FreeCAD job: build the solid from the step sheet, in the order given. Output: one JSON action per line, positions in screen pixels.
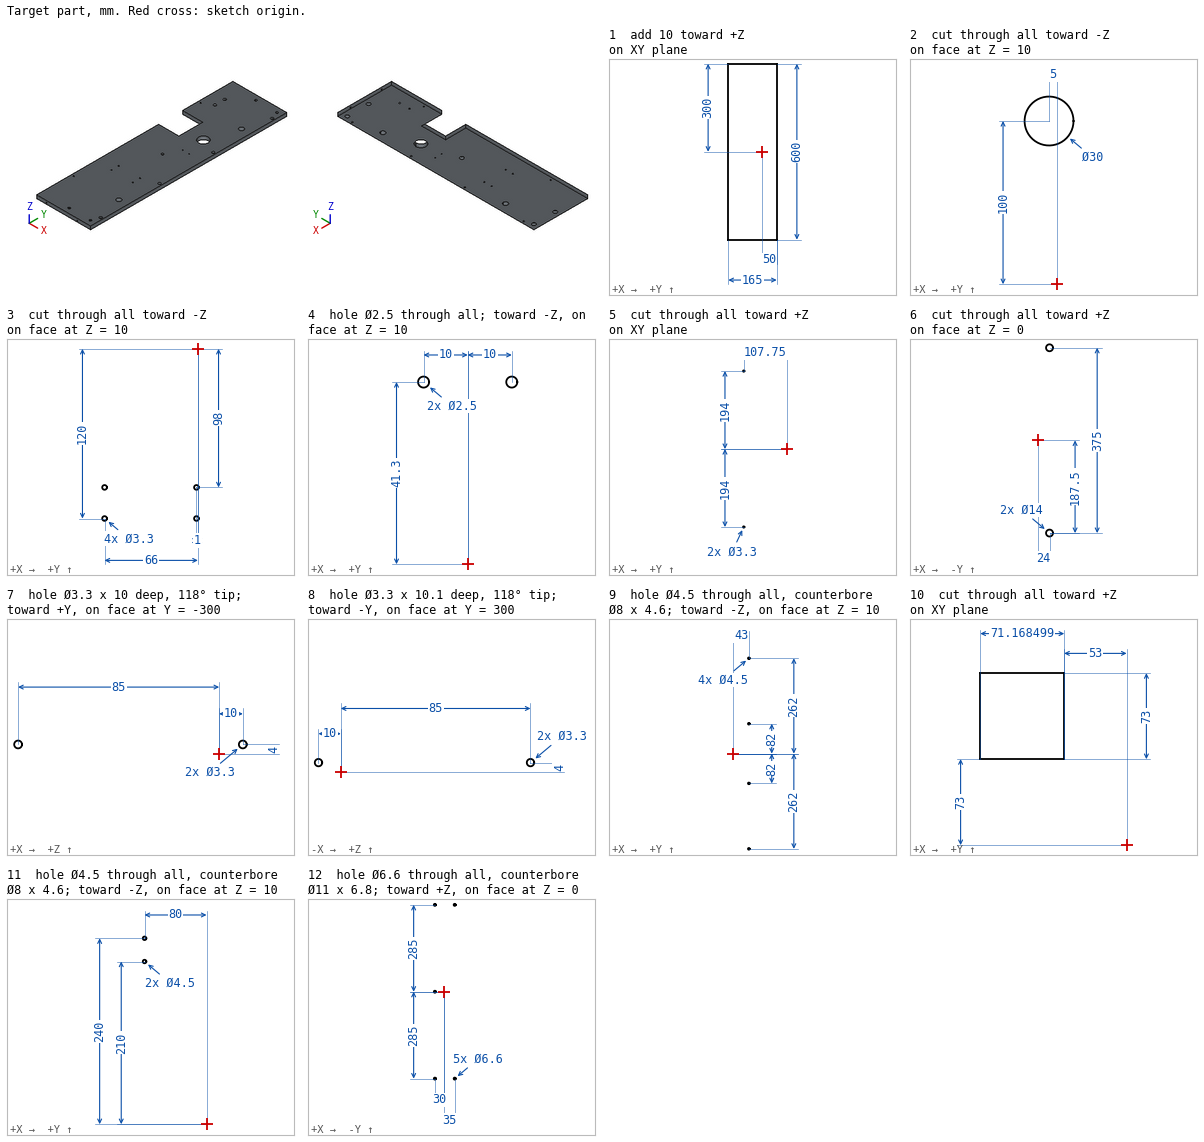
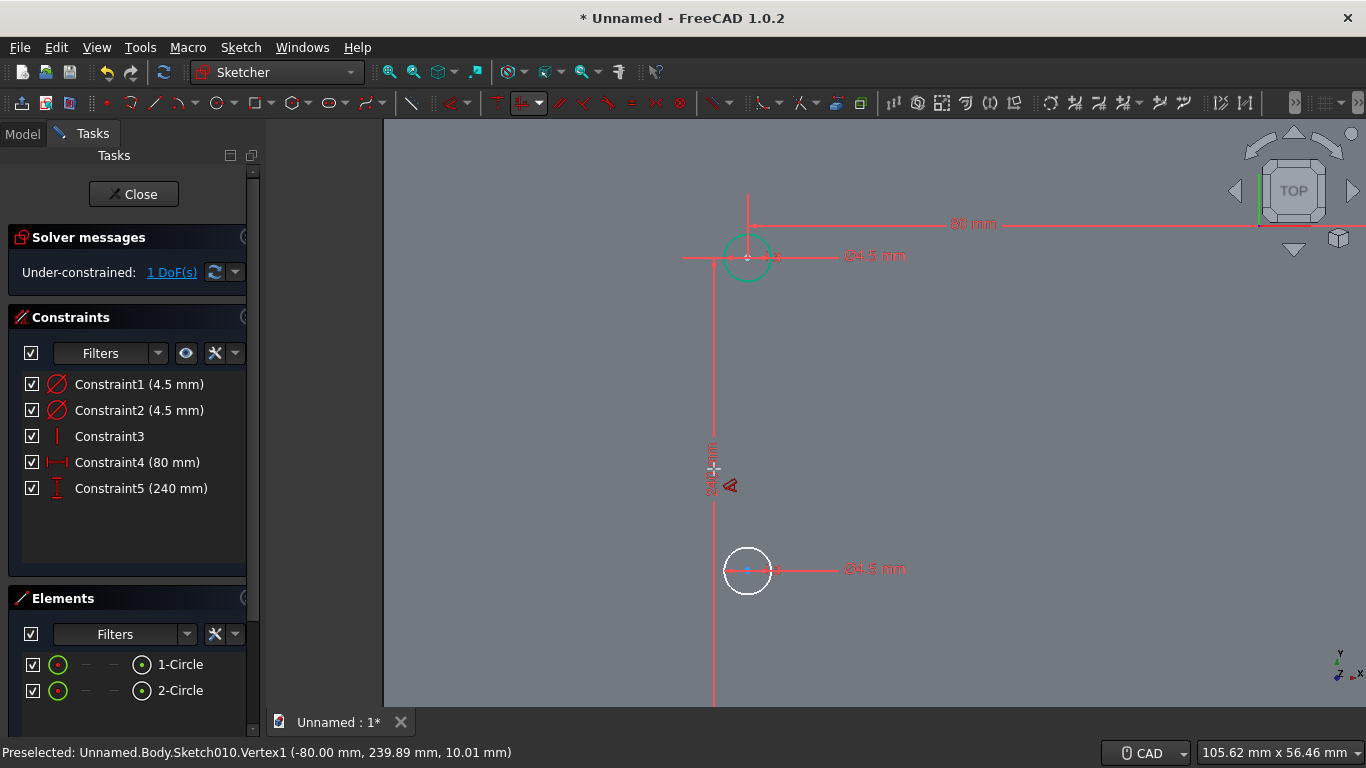
{"action": "left_click", "coordinate": [748, 571]}
{"action": "left_click", "coordinate": [714, 625]}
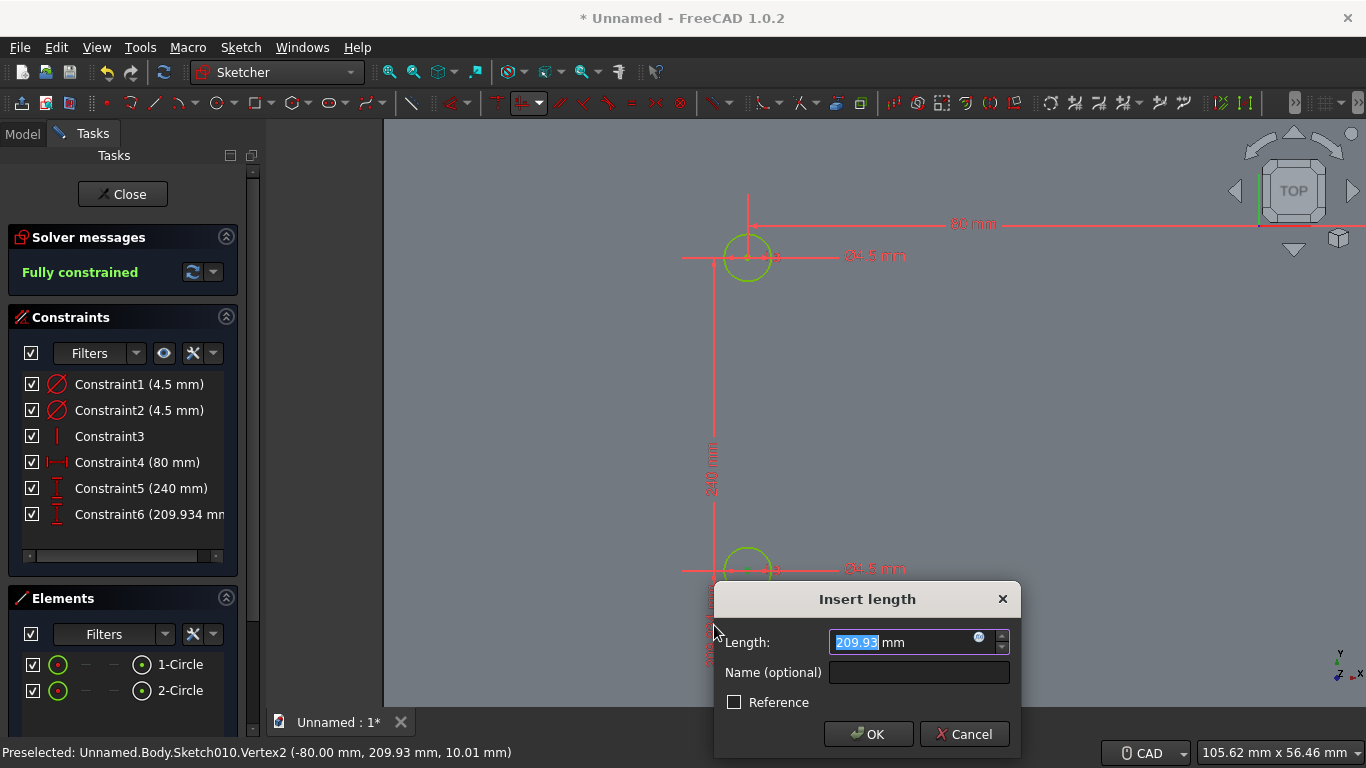
{"action": "type", "text": "210"}
{"action": "key", "text": "Return"}
{"action": "key", "text": "Escape"}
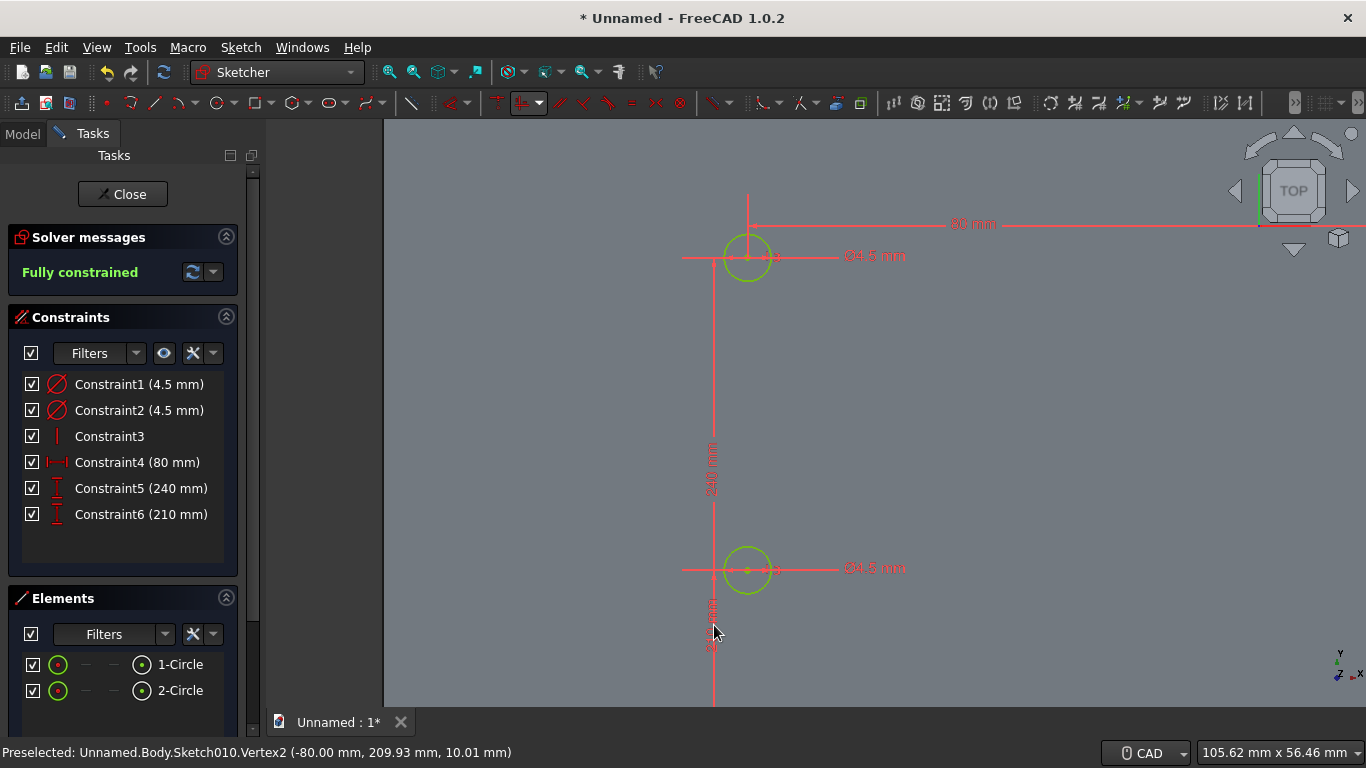
{"action": "left_click", "coordinate": [123, 194]}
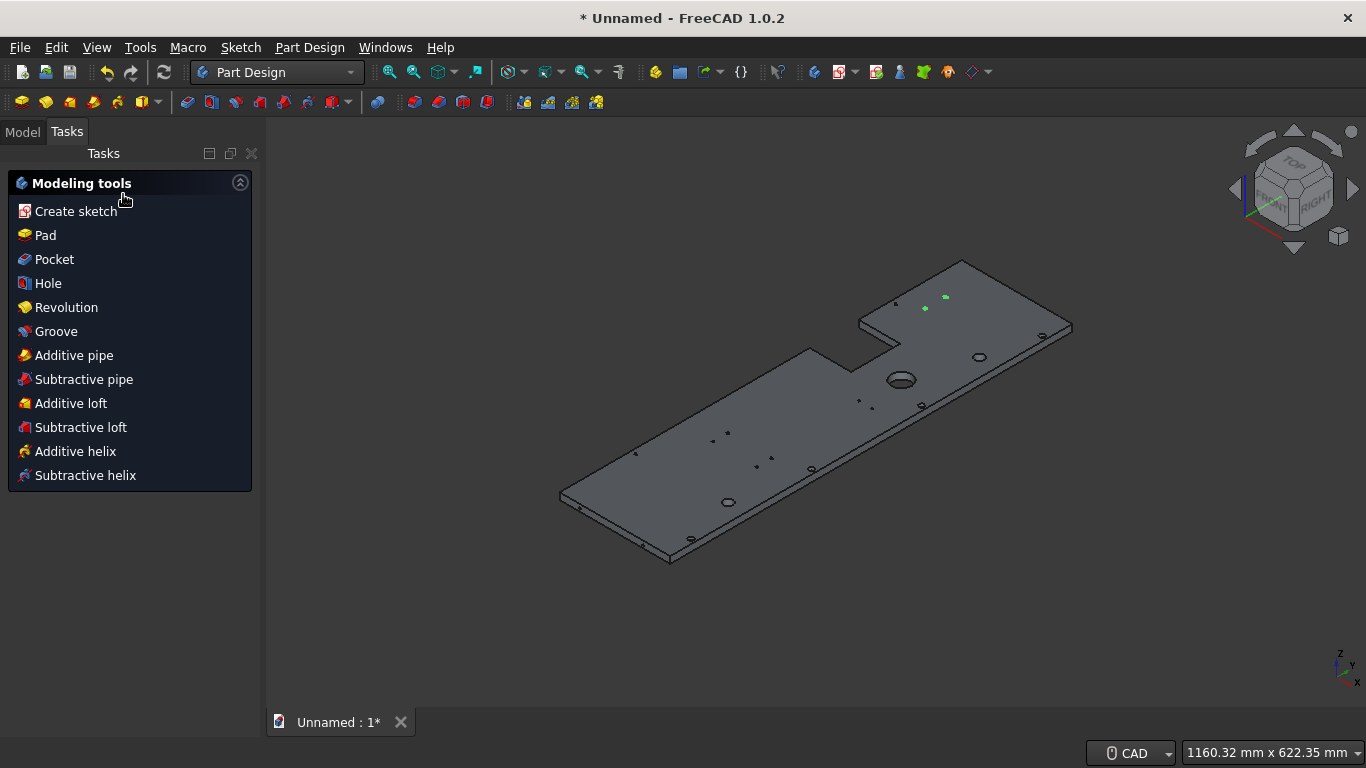
{"action": "left_click", "coordinate": [212, 102]}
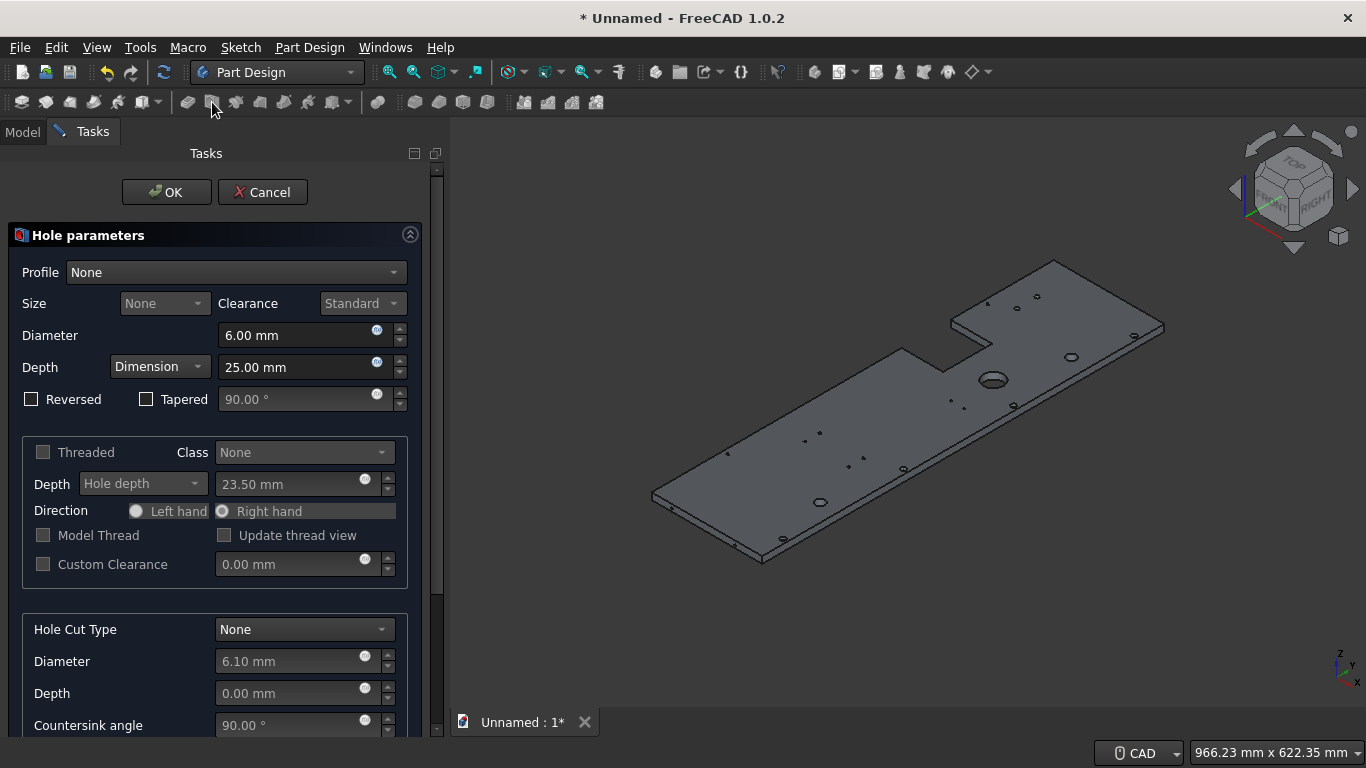
{"action": "triple_click", "coordinate": [305, 335]}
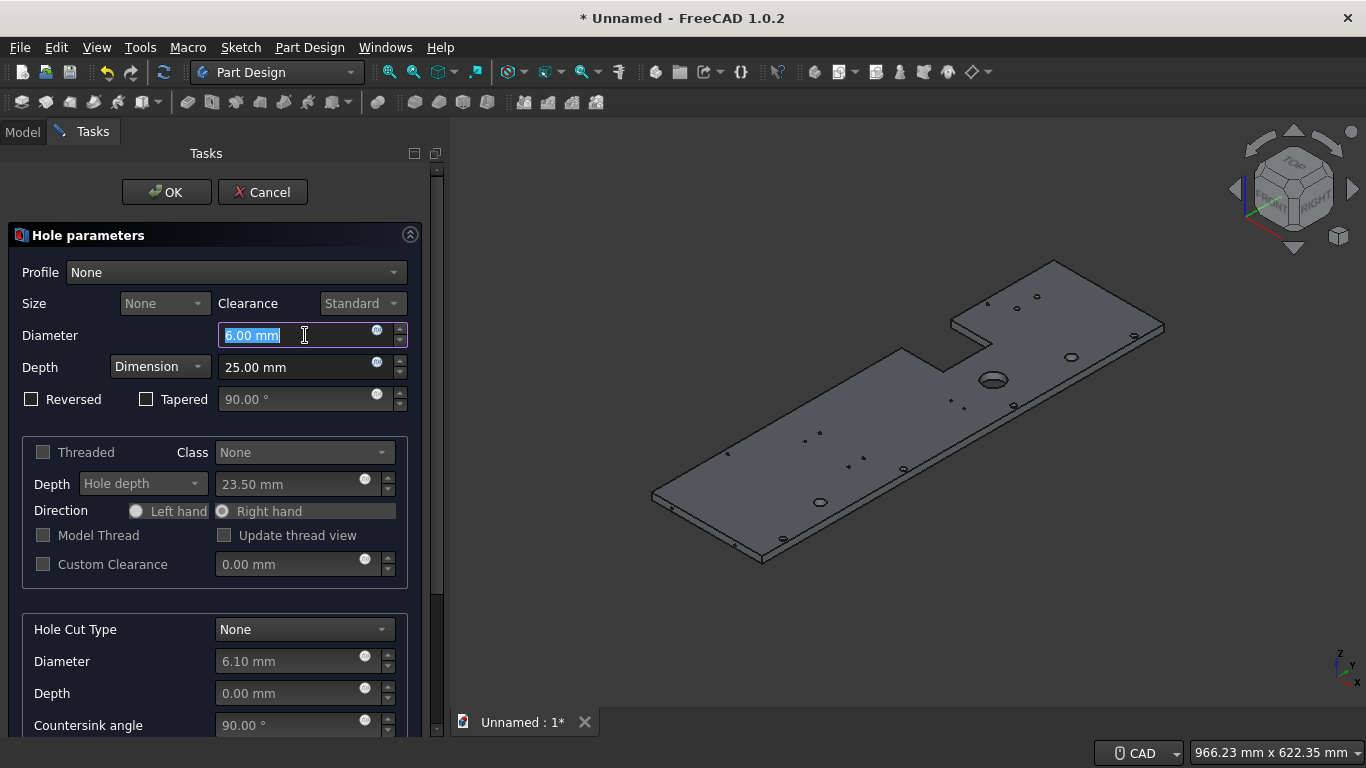
{"action": "type", "text": "4.5"}
{"action": "key", "text": "Tab"}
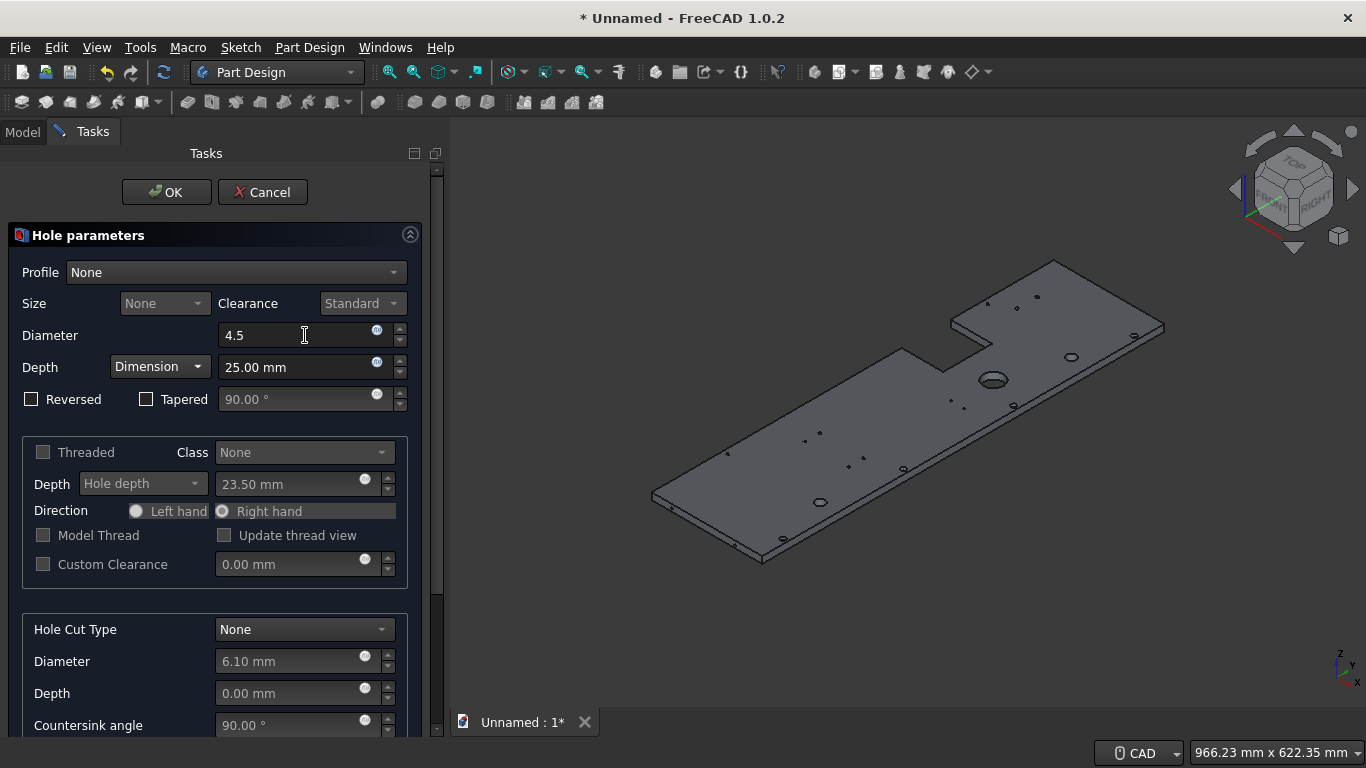
{"action": "left_click", "coordinate": [161, 366]}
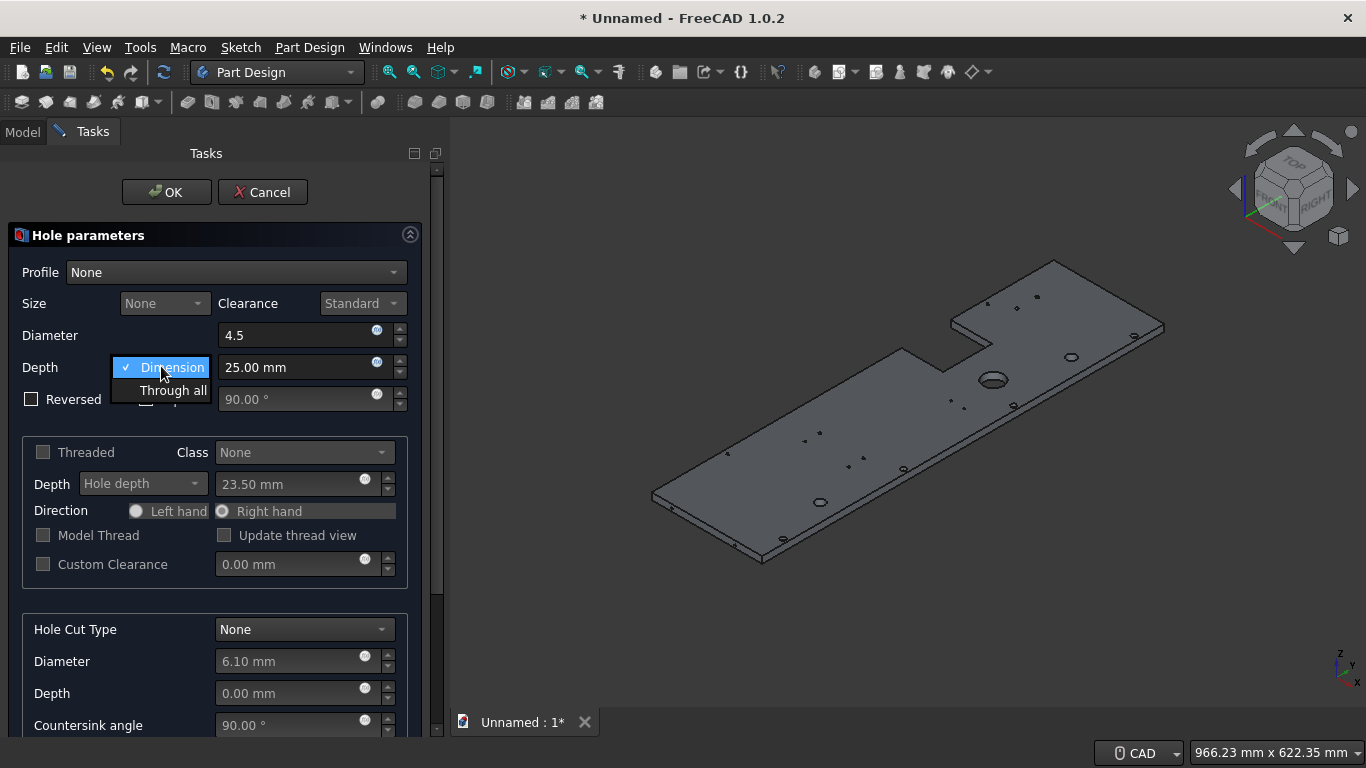
{"action": "left_click", "coordinate": [160, 390]}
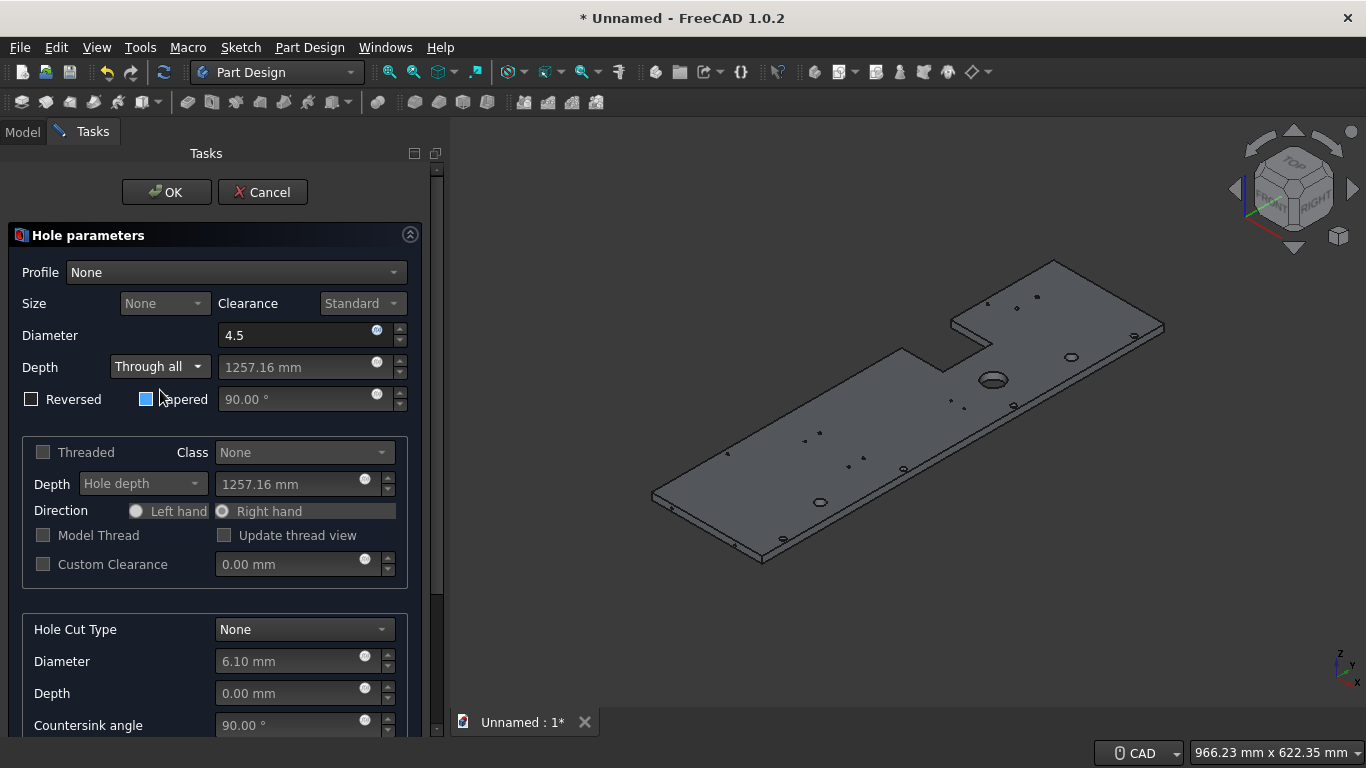
{"action": "left_click", "coordinate": [306, 630]}